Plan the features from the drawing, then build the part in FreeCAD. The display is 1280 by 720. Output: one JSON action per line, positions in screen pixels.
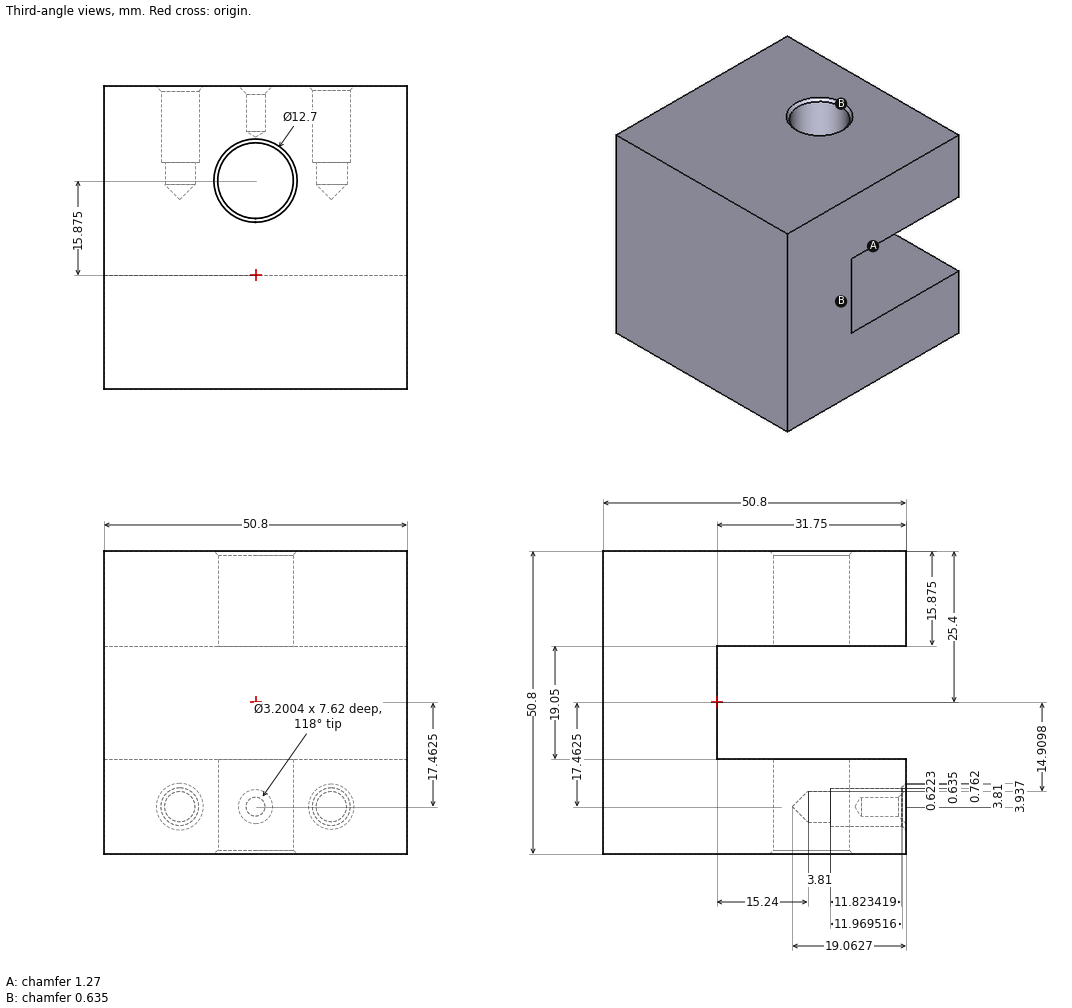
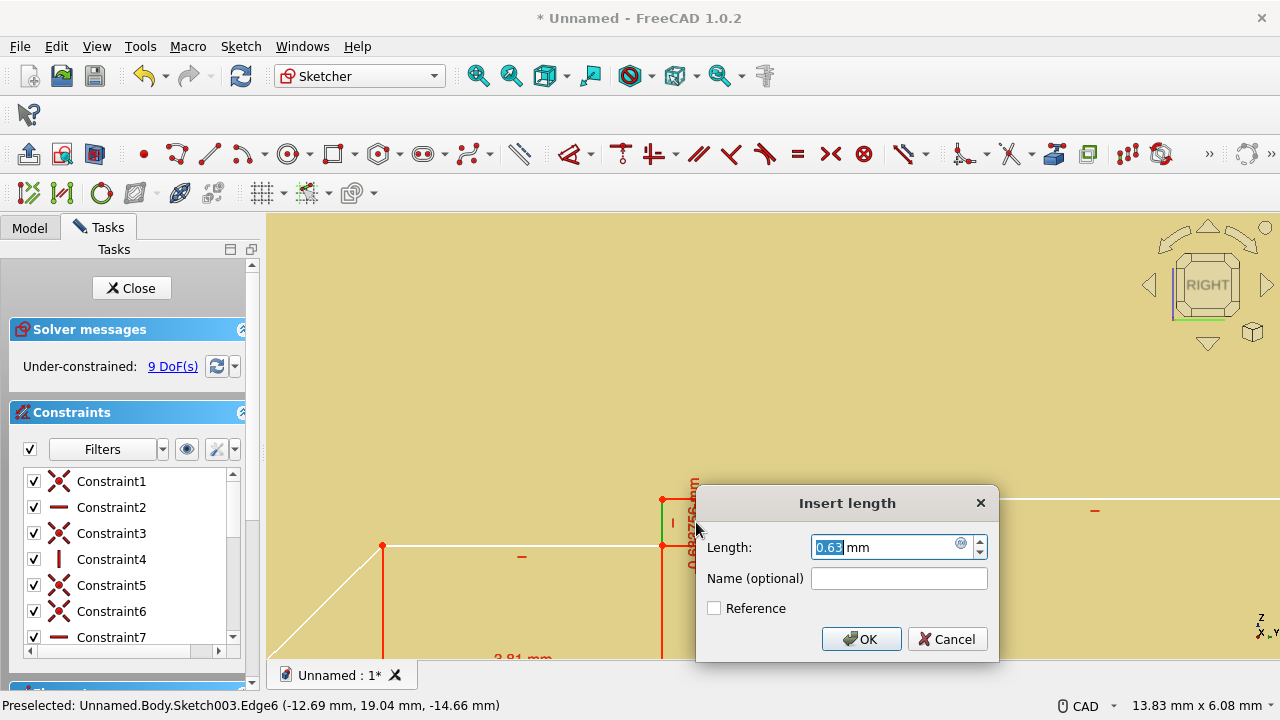
{"action": "type", "text": "0.6223"}
{"action": "key", "text": "Return"}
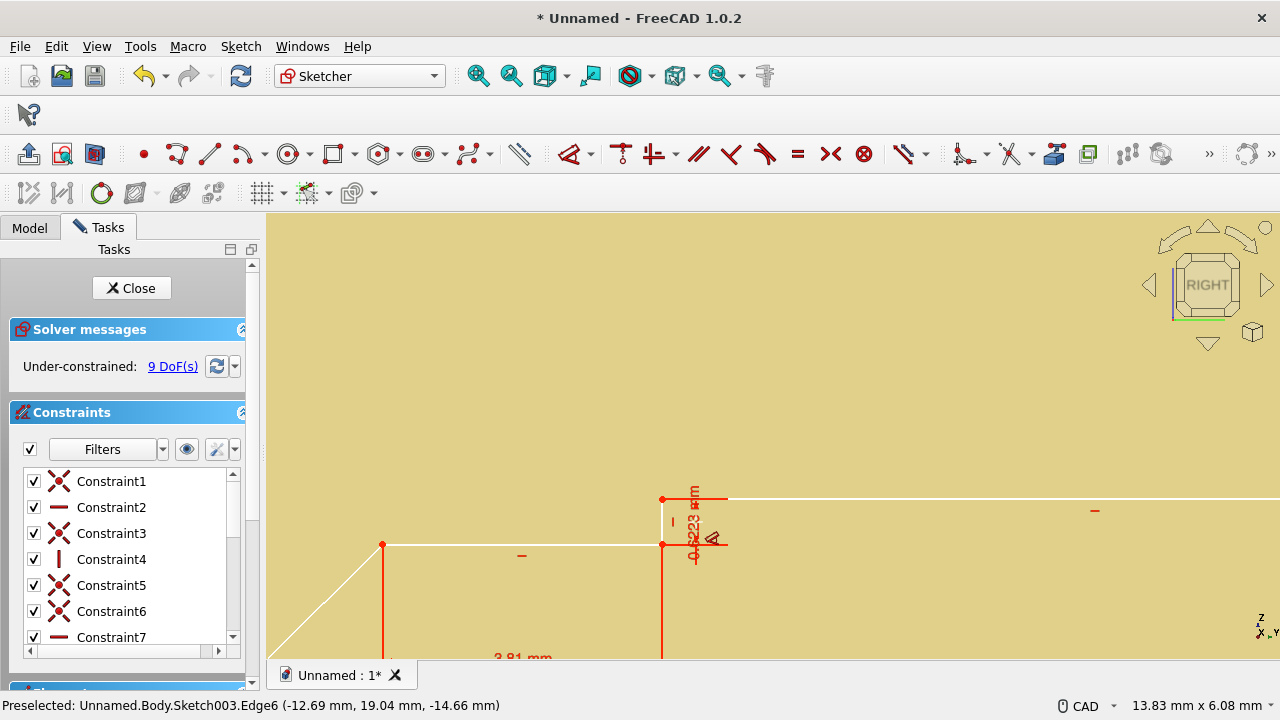
{"action": "scroll", "coordinate": [774, 524], "scroll_direction": "down", "scroll_amount": 8}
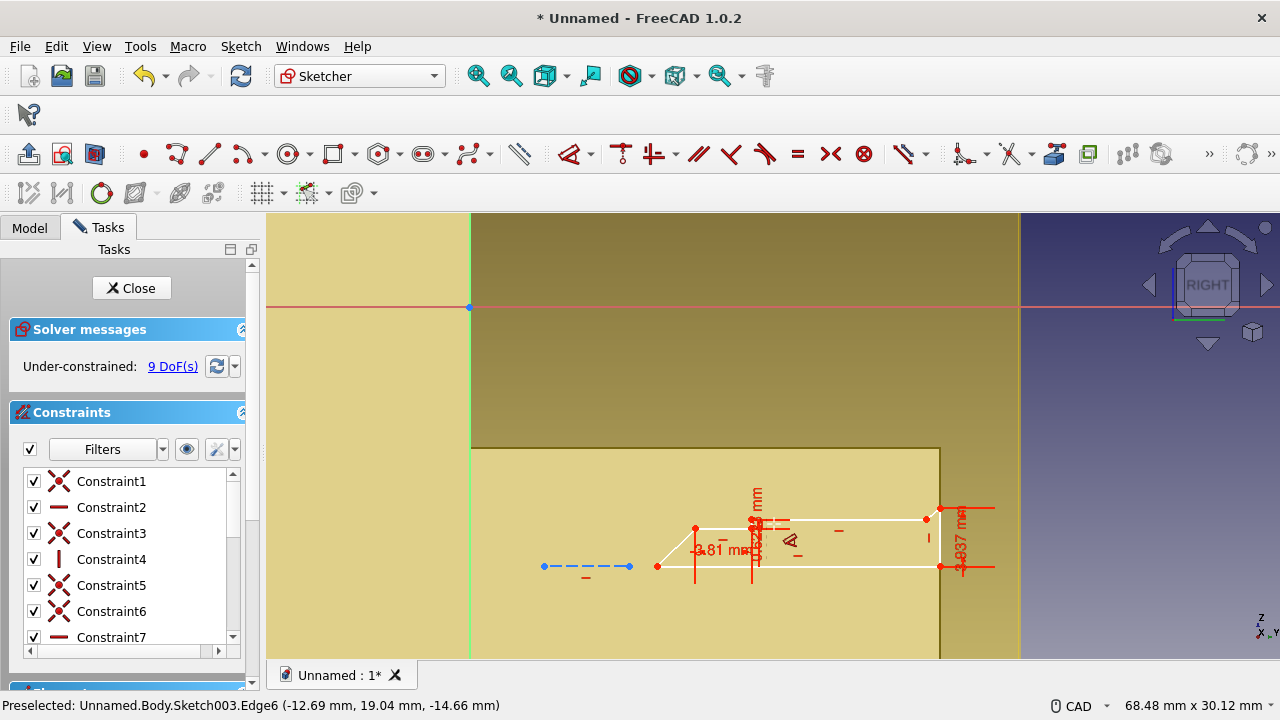
{"action": "left_click", "coordinate": [695, 529]}
{"action": "left_click", "coordinate": [583, 273]}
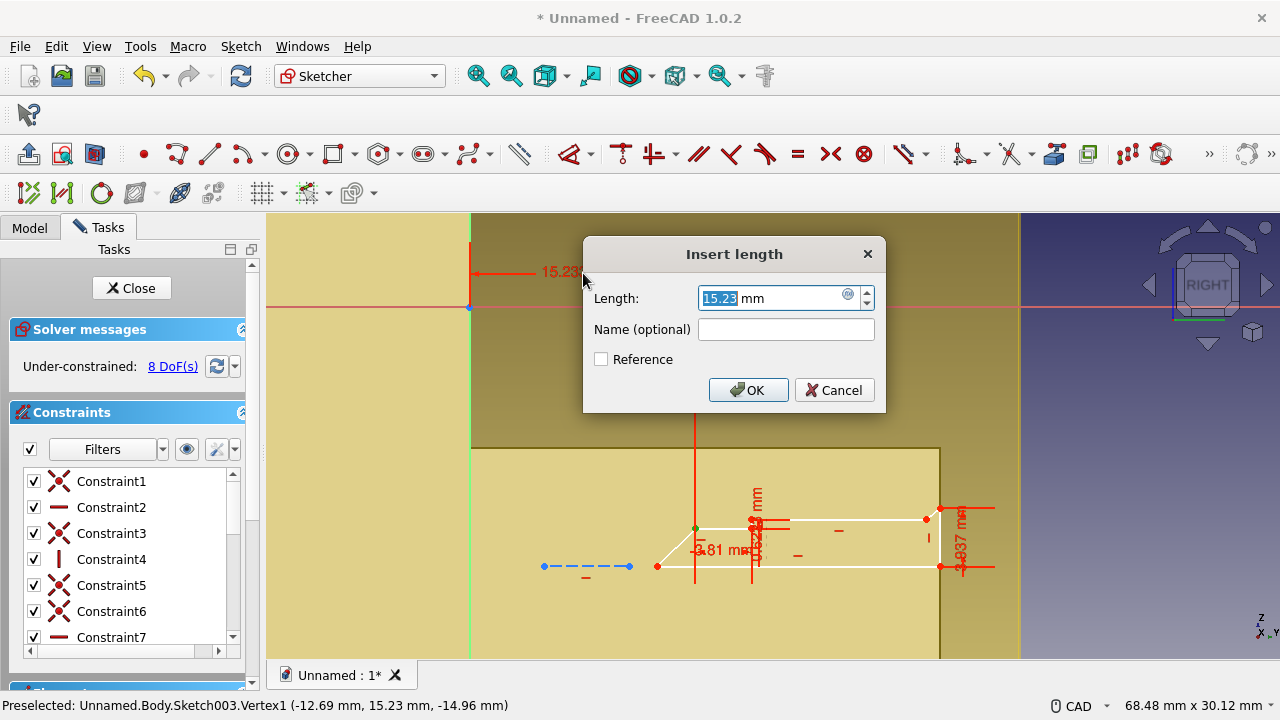
{"action": "type", "text": "15.24"}
{"action": "key", "text": "Return"}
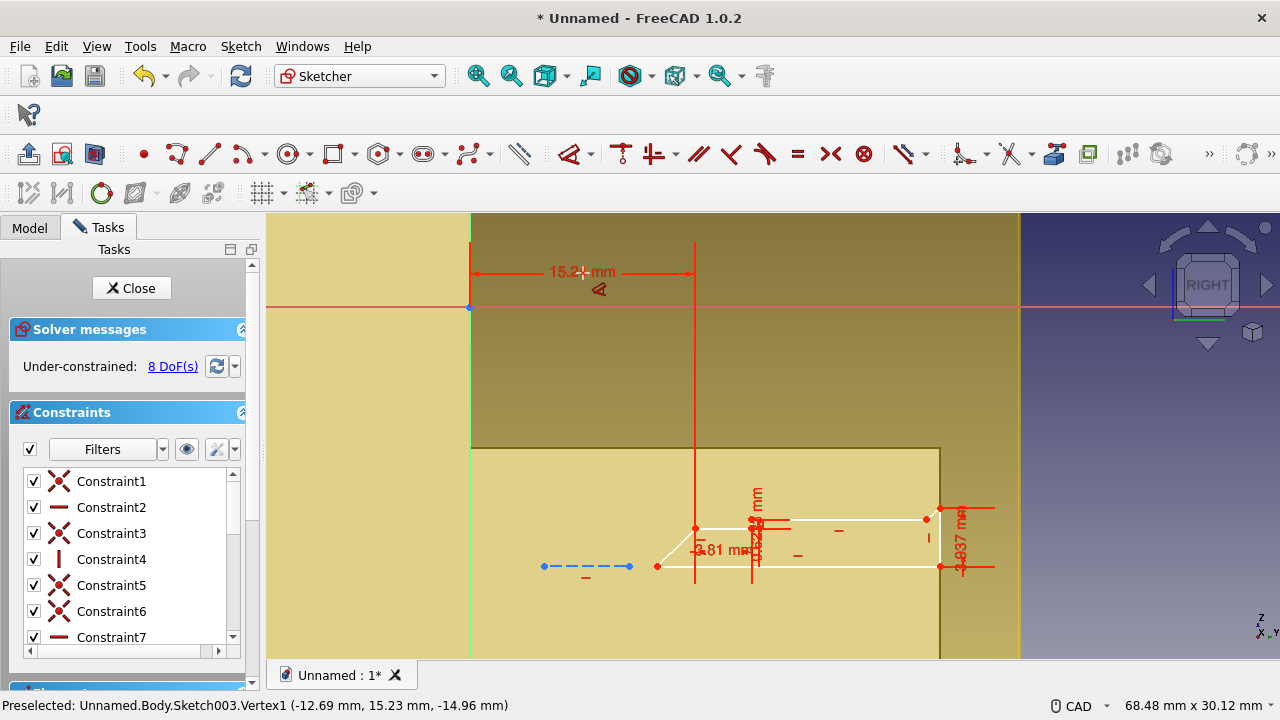
{"action": "left_click", "coordinate": [940, 567]}
{"action": "left_click", "coordinate": [705, 601]}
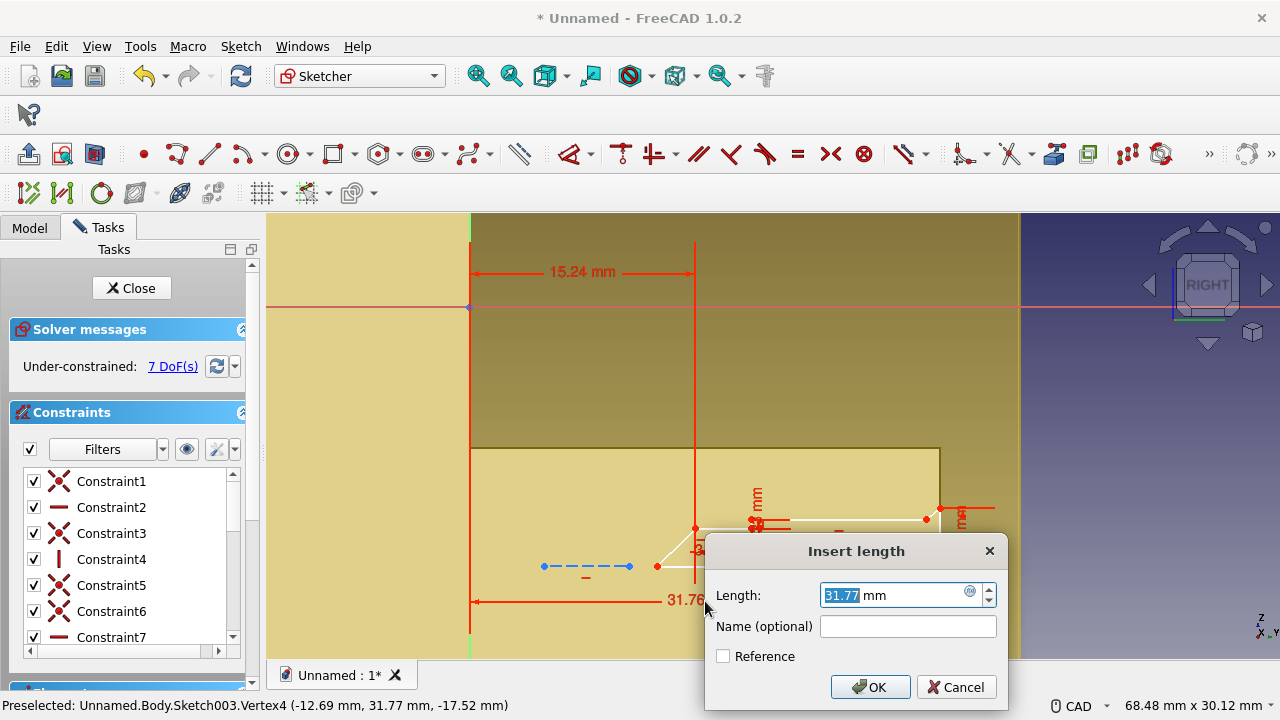
{"action": "type", "text": "31.75"}
{"action": "key", "text": "Return"}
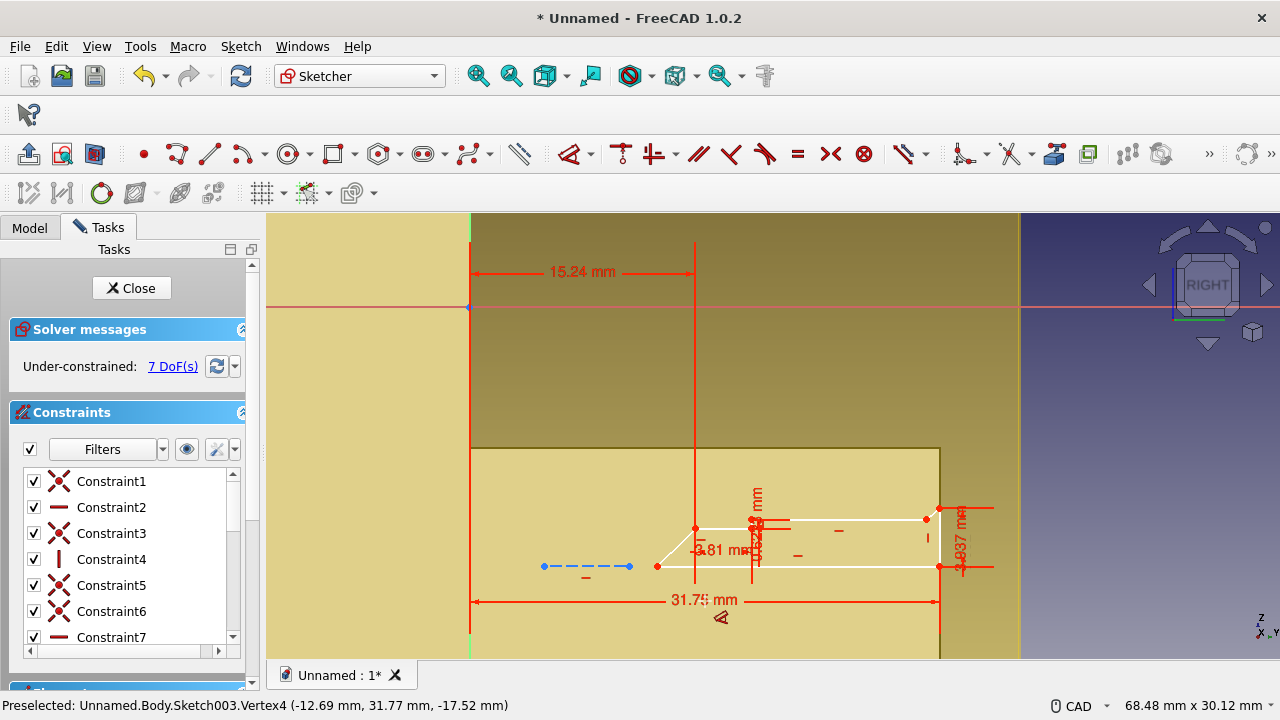
{"action": "scroll", "coordinate": [932, 515], "scroll_direction": "up", "scroll_amount": 7}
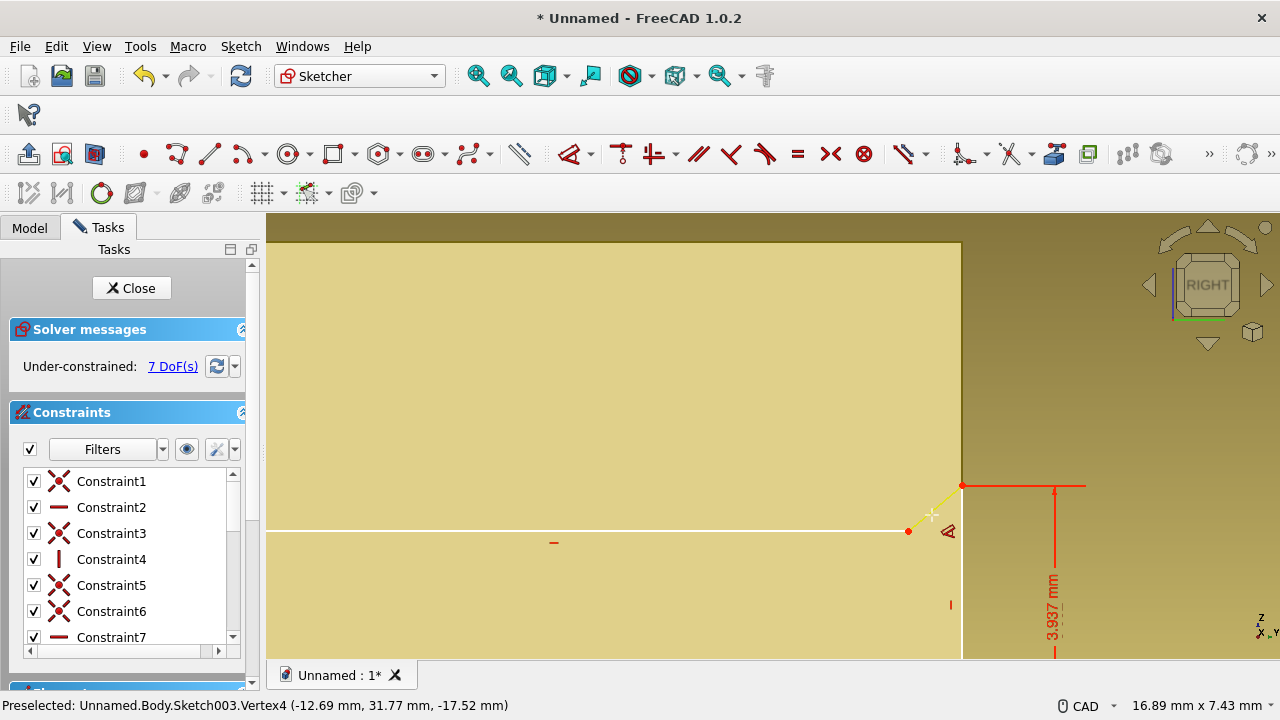
{"action": "left_click", "coordinate": [930, 513]}
{"action": "left_click", "coordinate": [996, 509]}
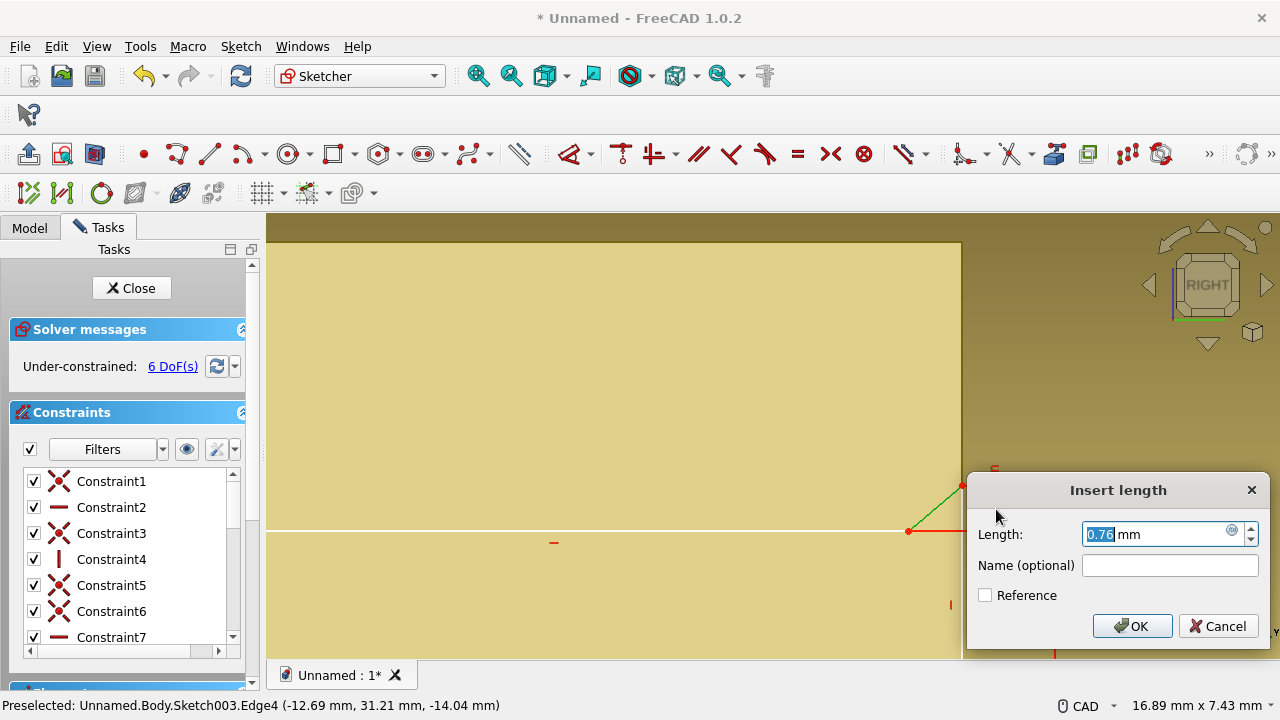
{"action": "type", "text": "0.762"}
{"action": "key", "text": "Return"}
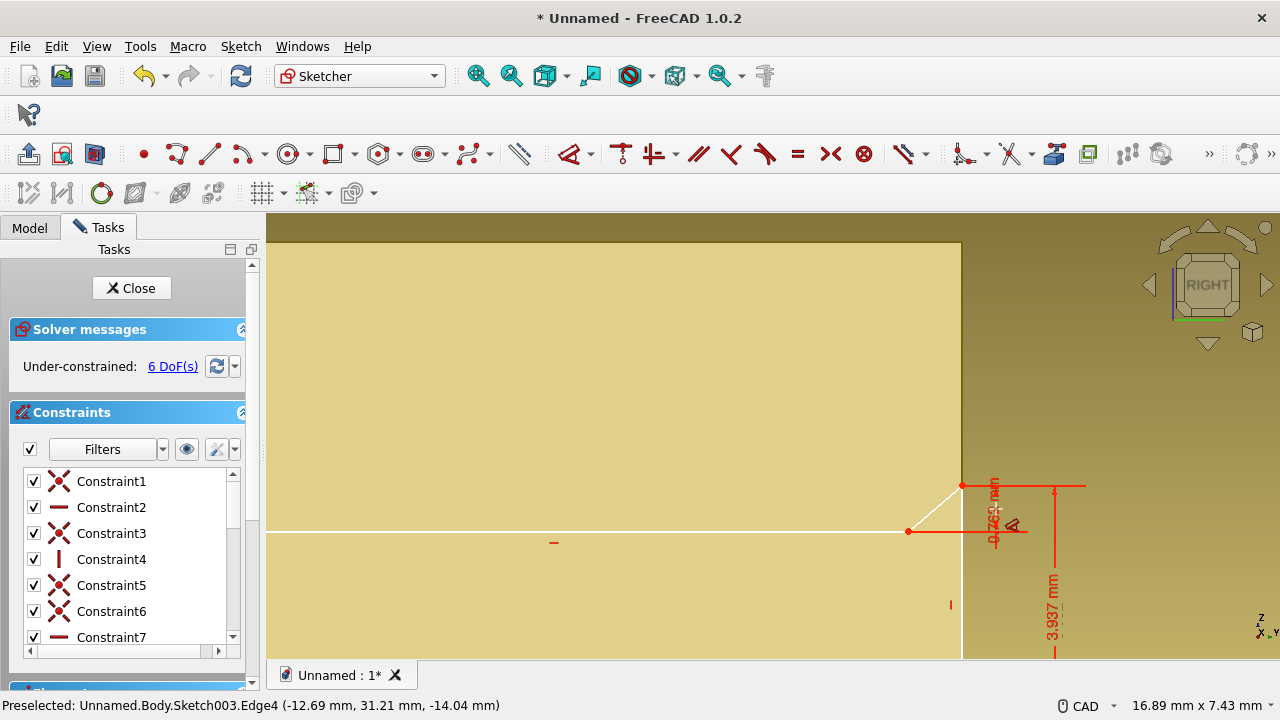
{"action": "scroll", "coordinate": [932, 515], "scroll_direction": "down", "scroll_amount": 7}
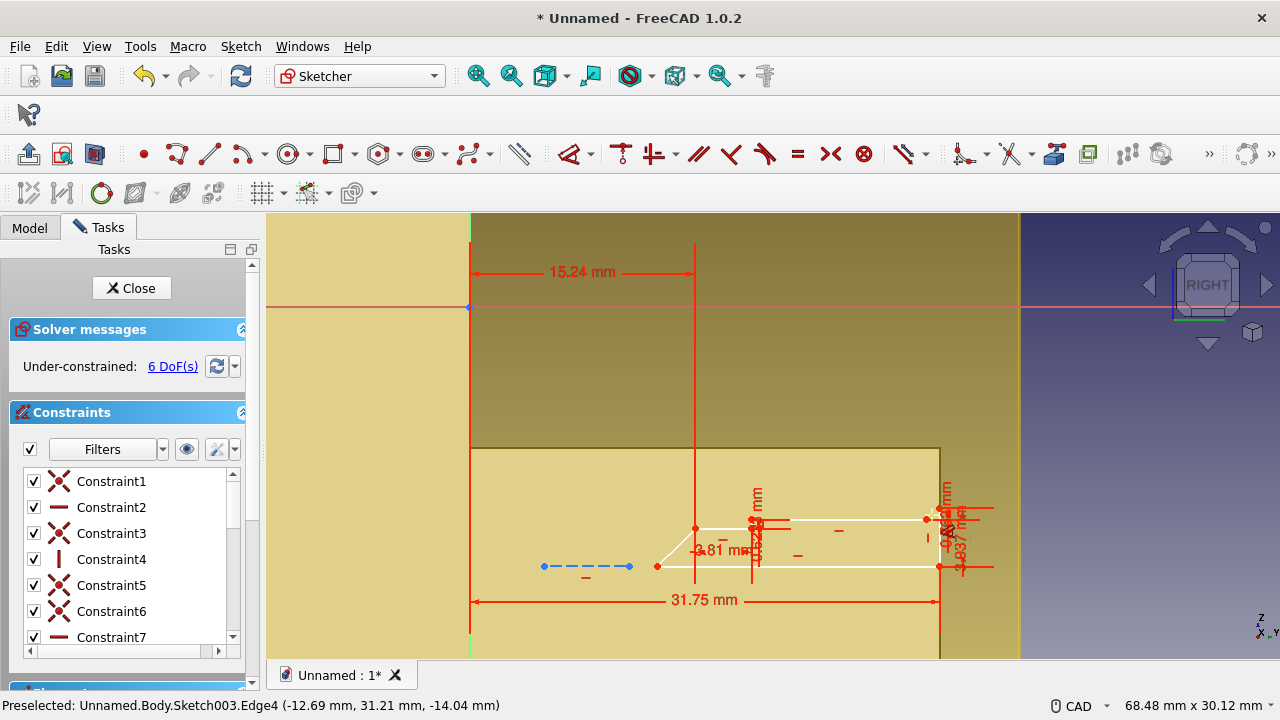
{"action": "left_click", "coordinate": [742, 567]}
{"action": "left_click", "coordinate": [799, 601]}